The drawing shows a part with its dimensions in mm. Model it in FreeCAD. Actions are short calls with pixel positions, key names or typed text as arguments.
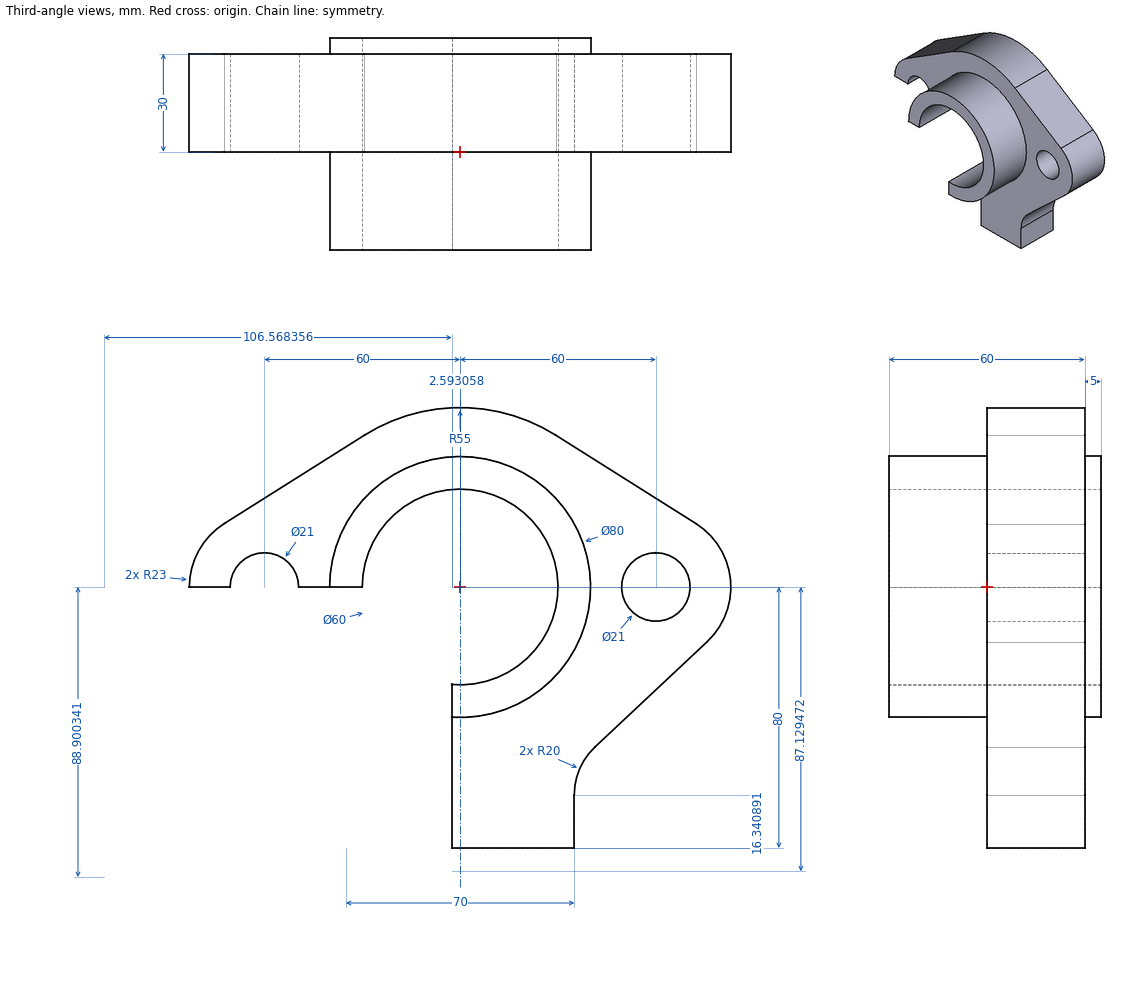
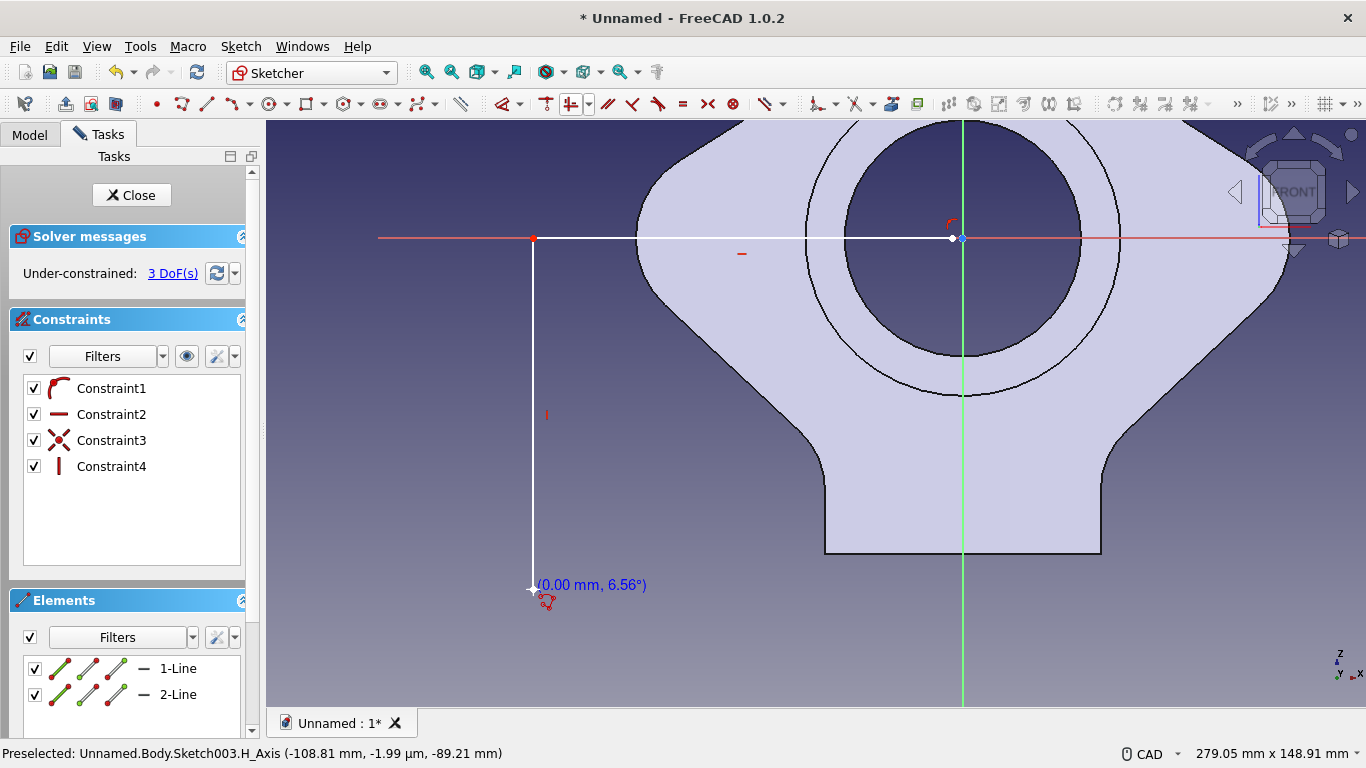
scroll(953, 582, up, 3)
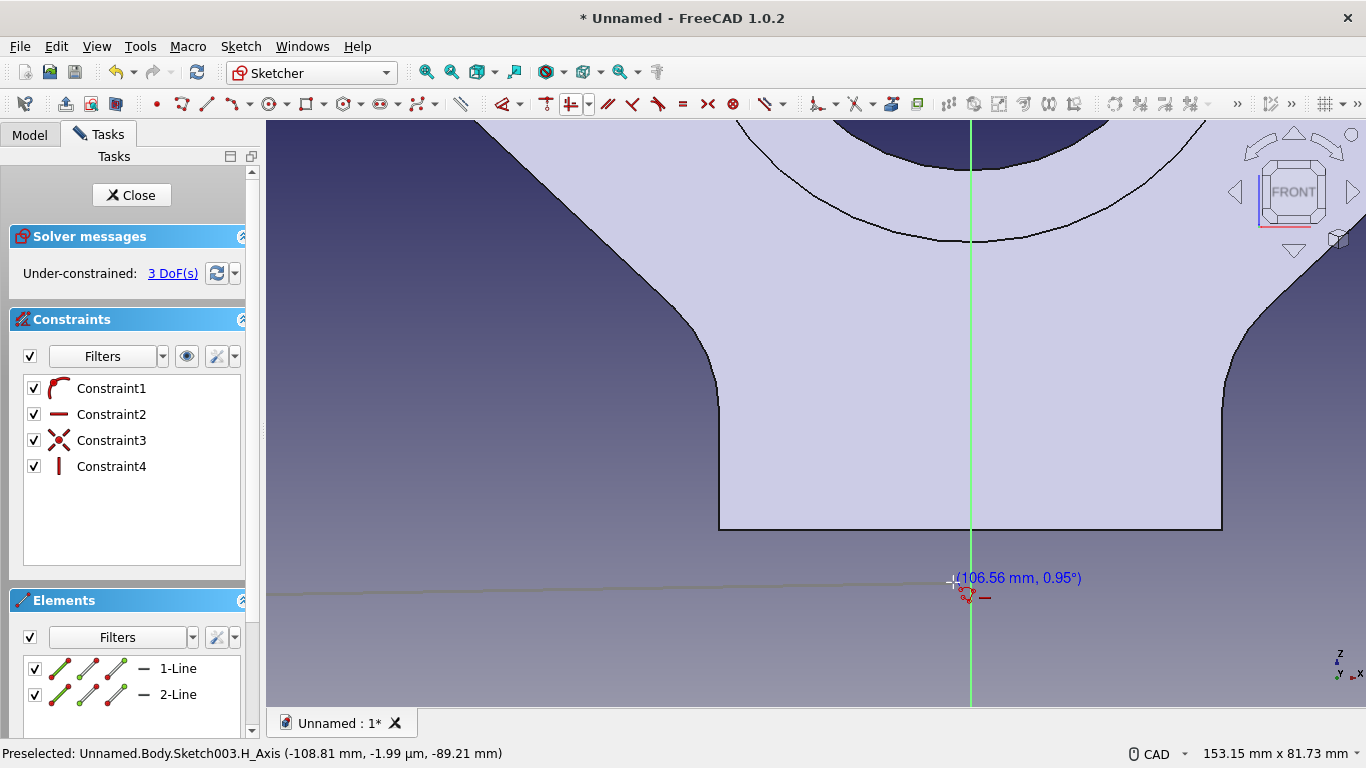
click(952, 558)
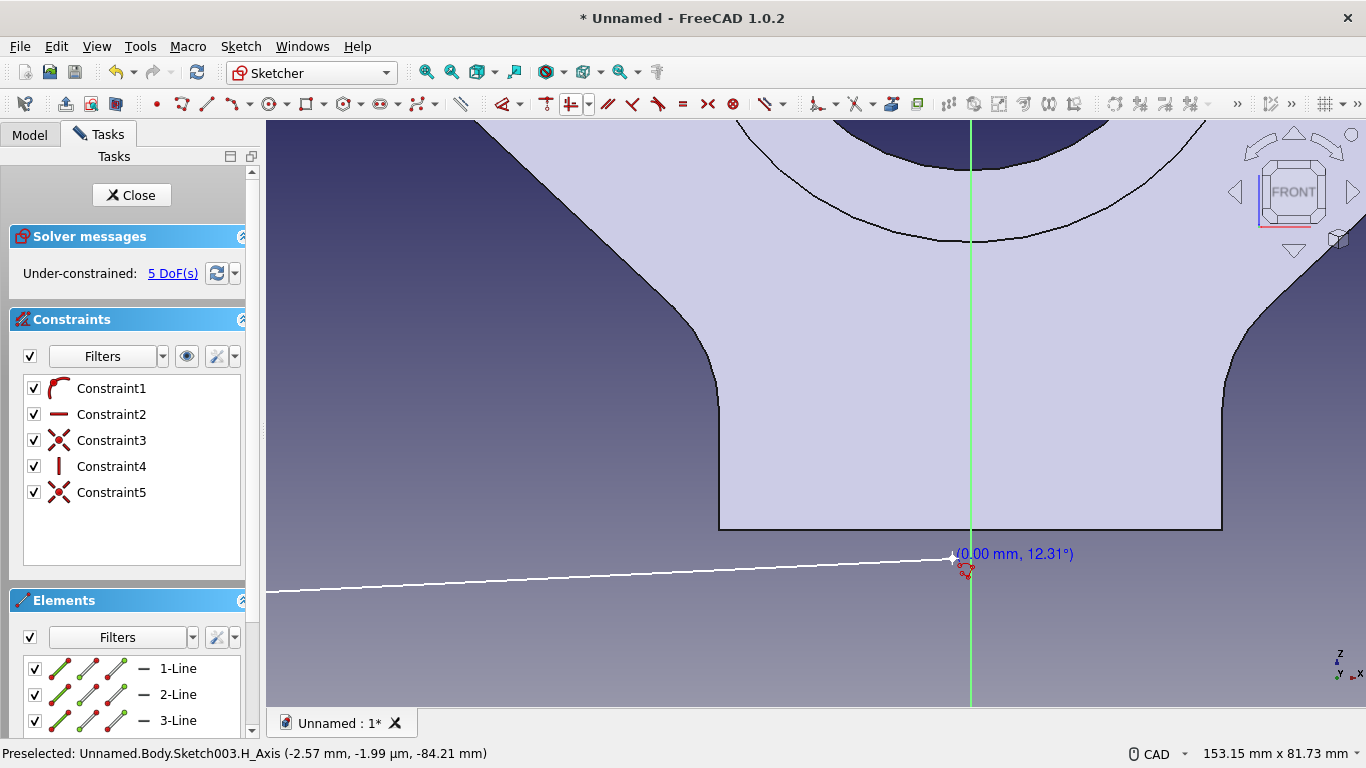
scroll(953, 583, down, 3)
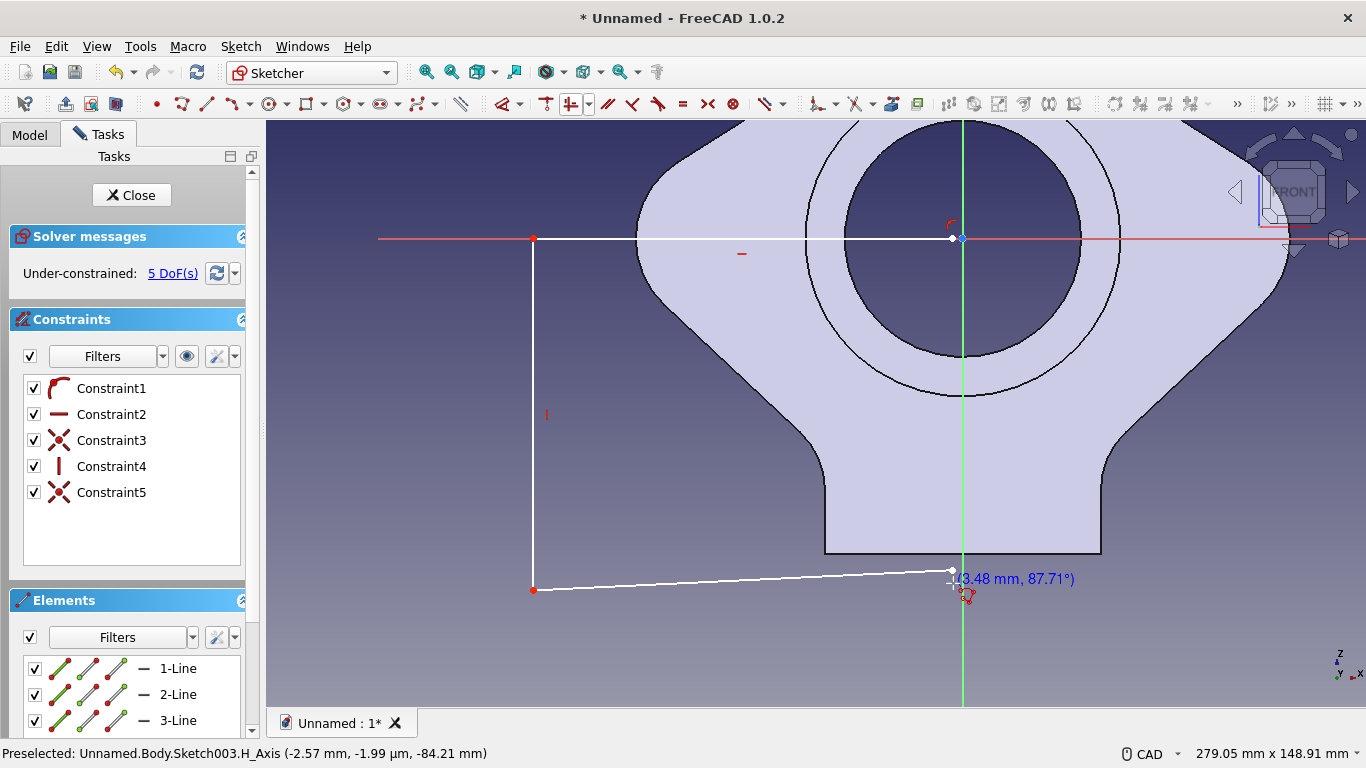
scroll(953, 239, up, 3)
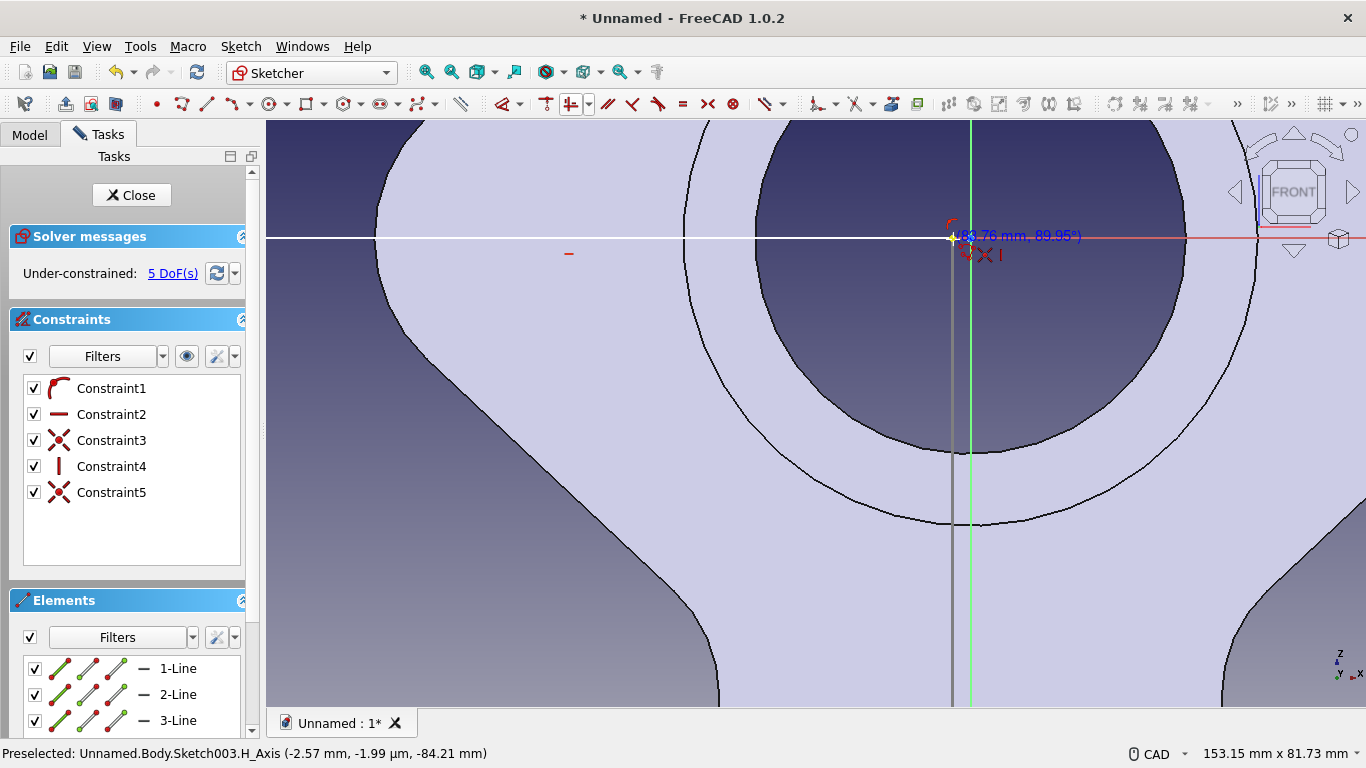
click(952, 238)
key(Escape)
key(Escape)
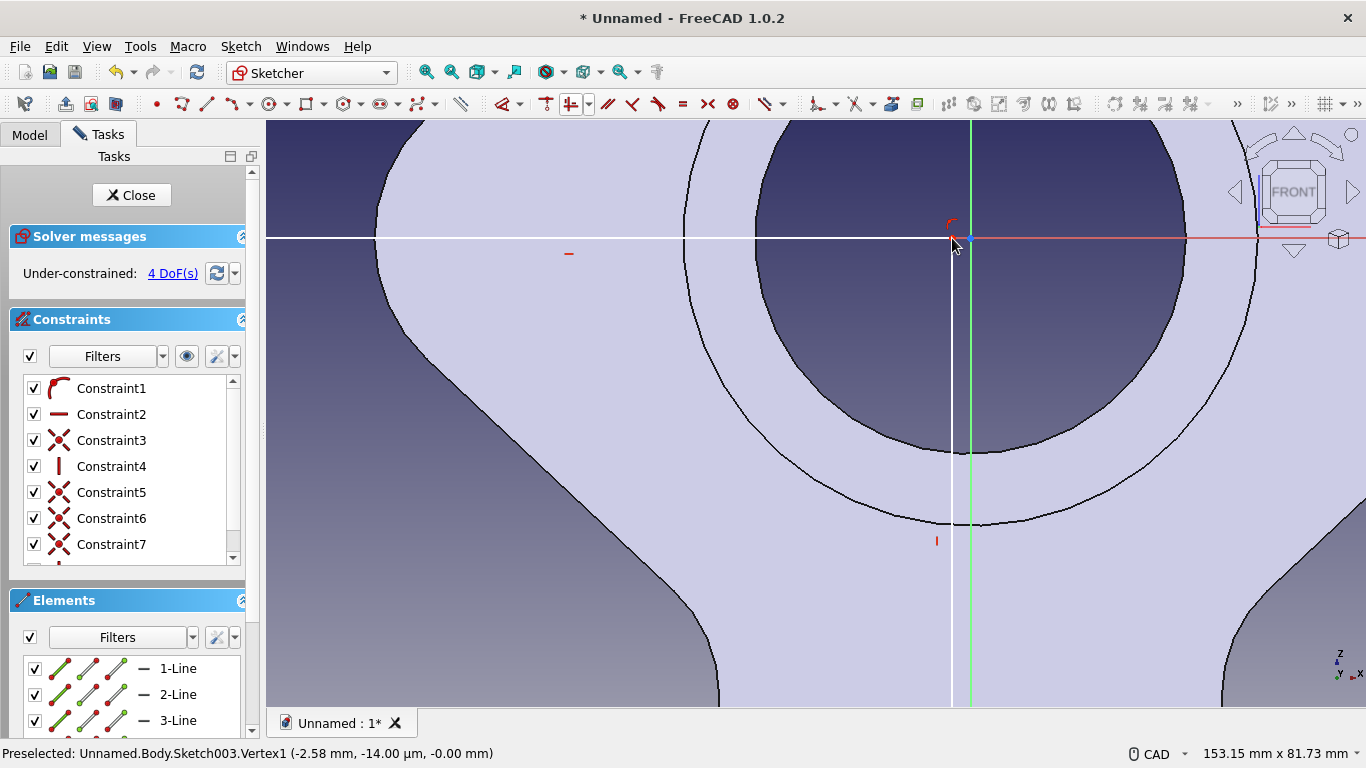
click(502, 104)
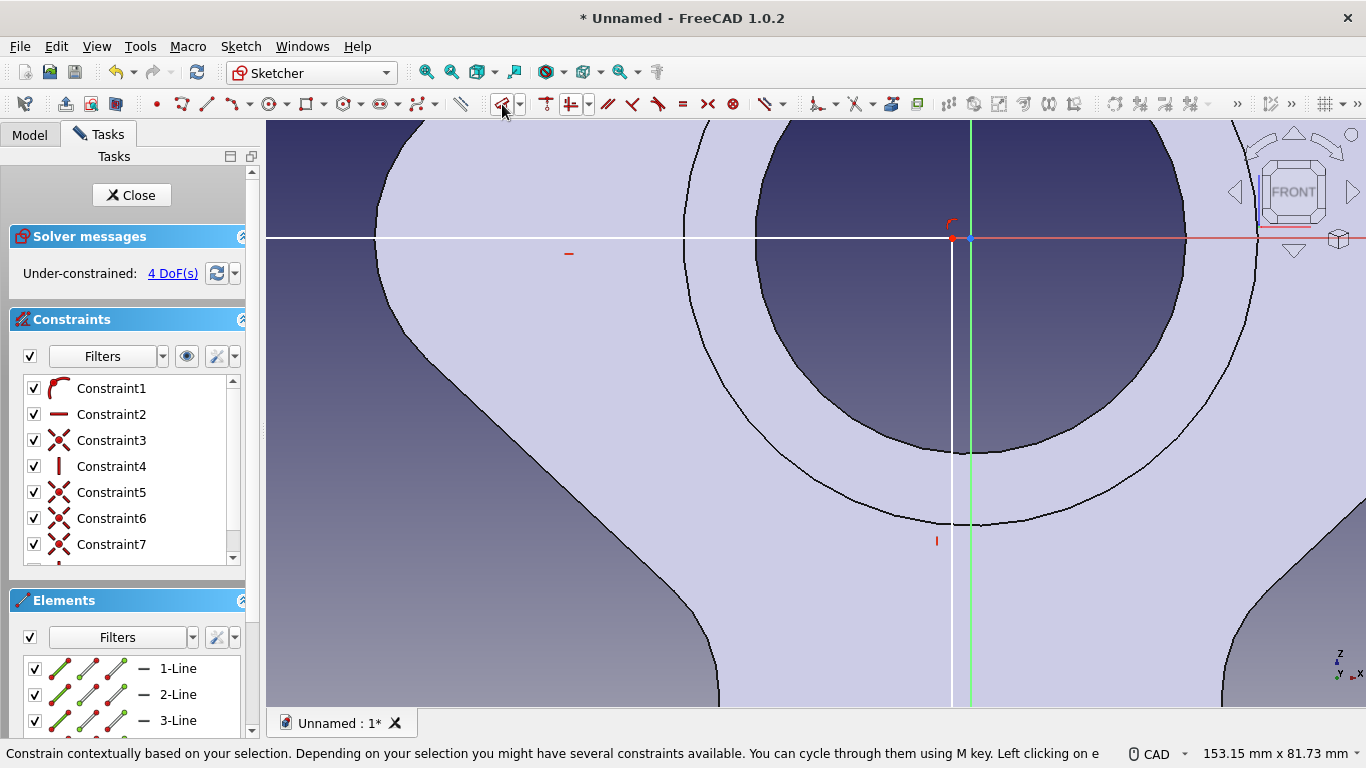
scroll(953, 238, down, 3)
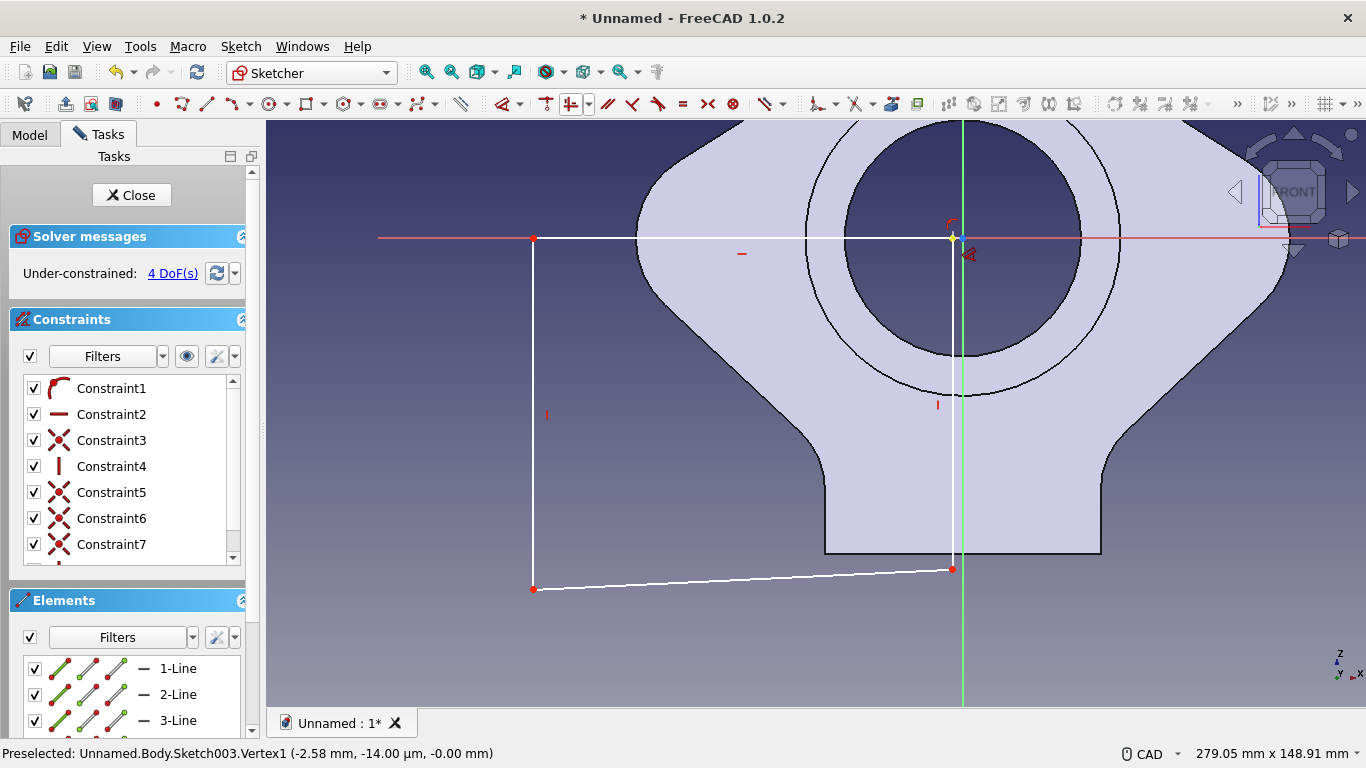
click(533, 344)
click(499, 414)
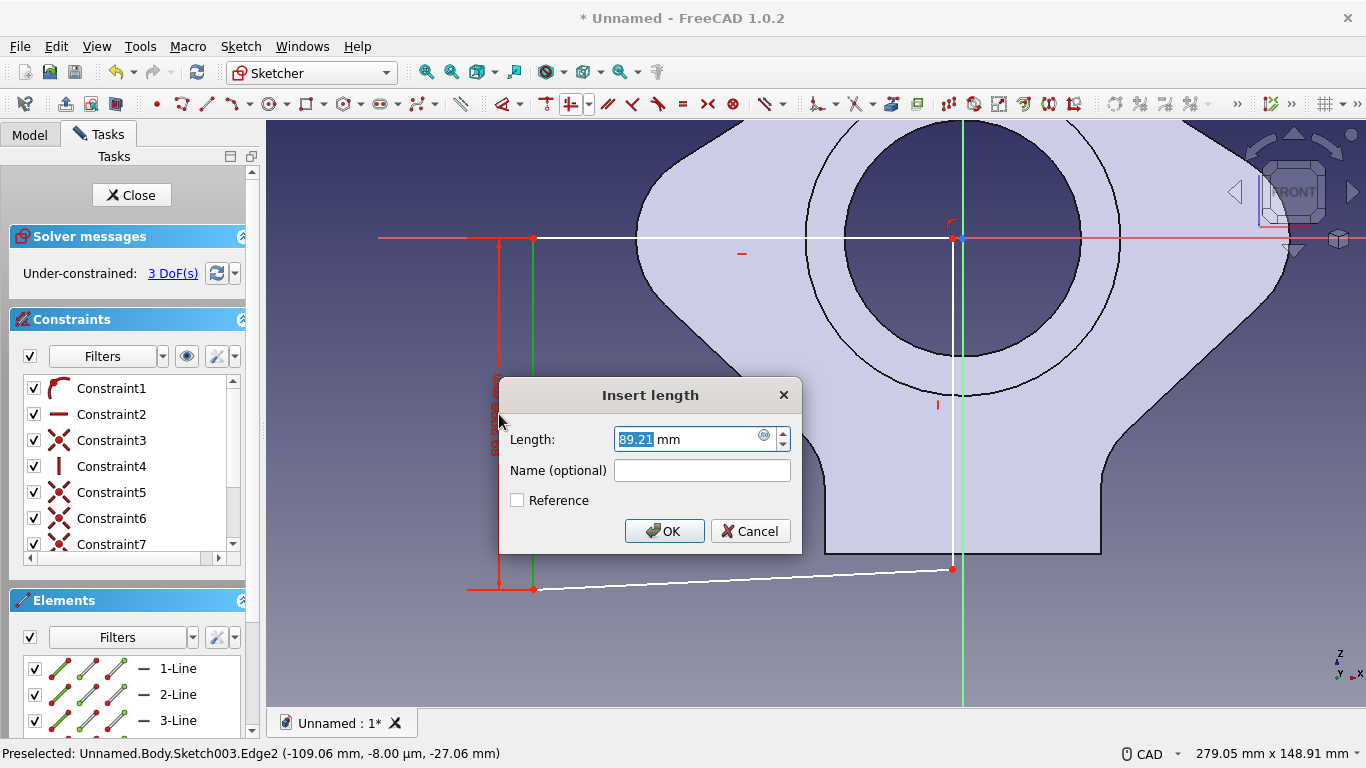
text(88.900341)
key(Return)